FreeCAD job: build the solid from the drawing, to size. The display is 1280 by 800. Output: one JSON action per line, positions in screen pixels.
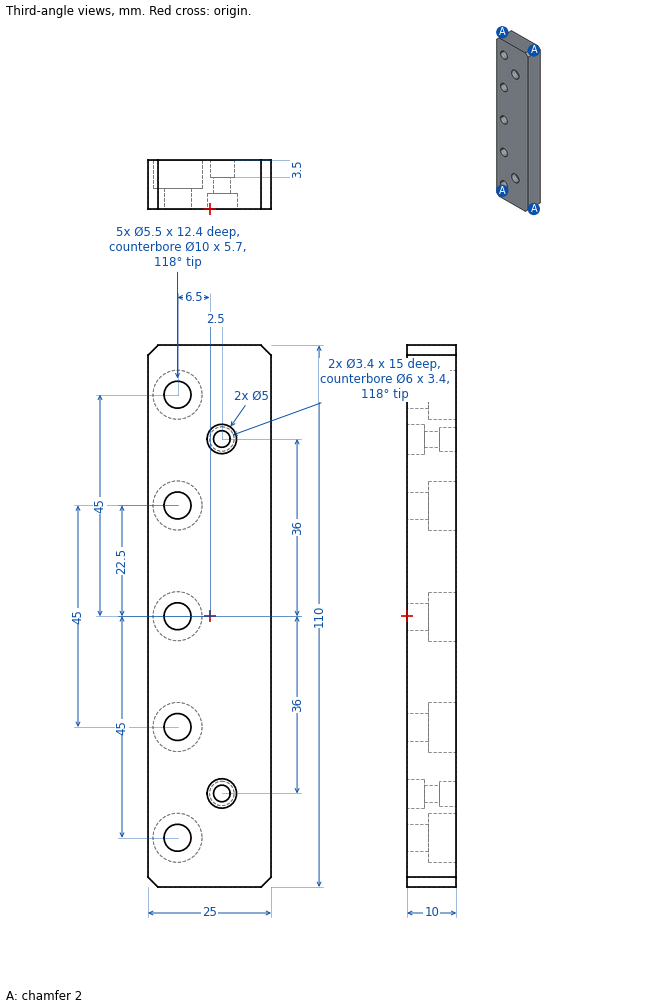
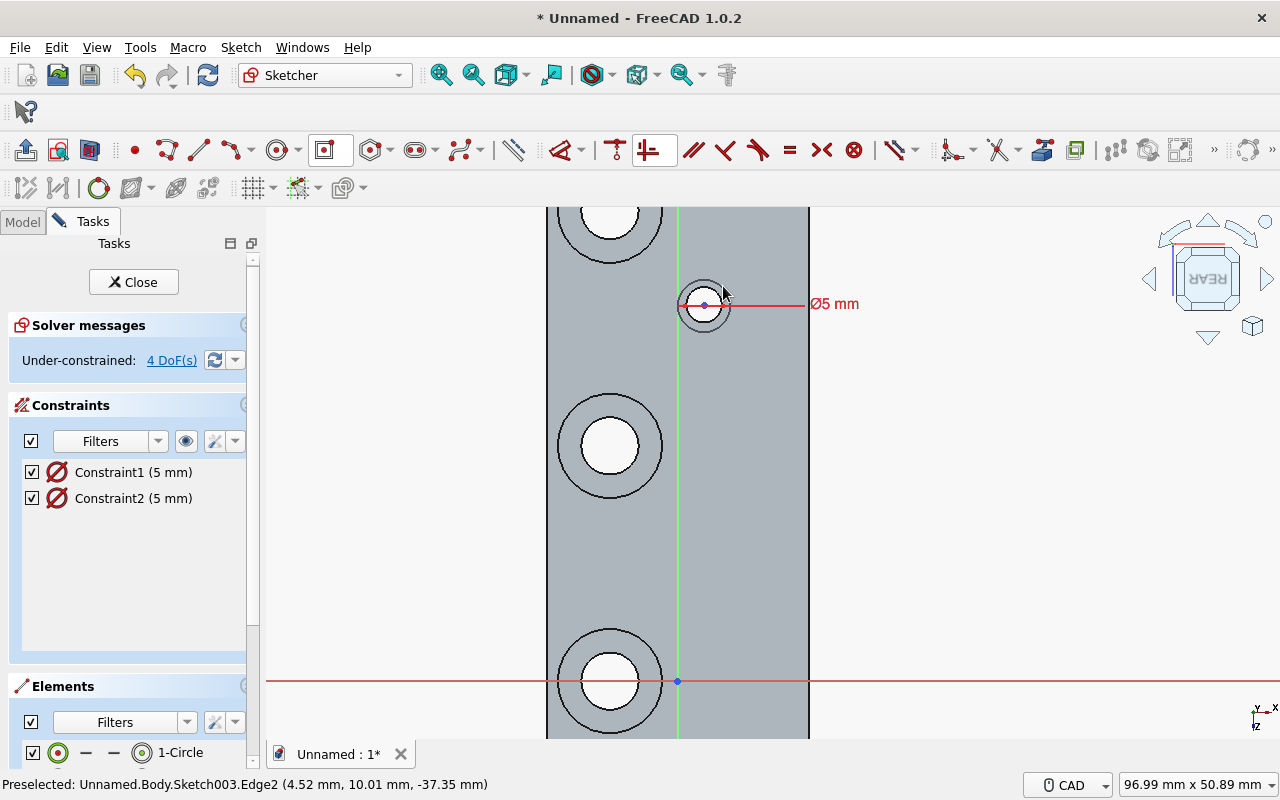
{"action": "scroll", "coordinate": [705, 303], "scroll_direction": "down", "scroll_amount": 4}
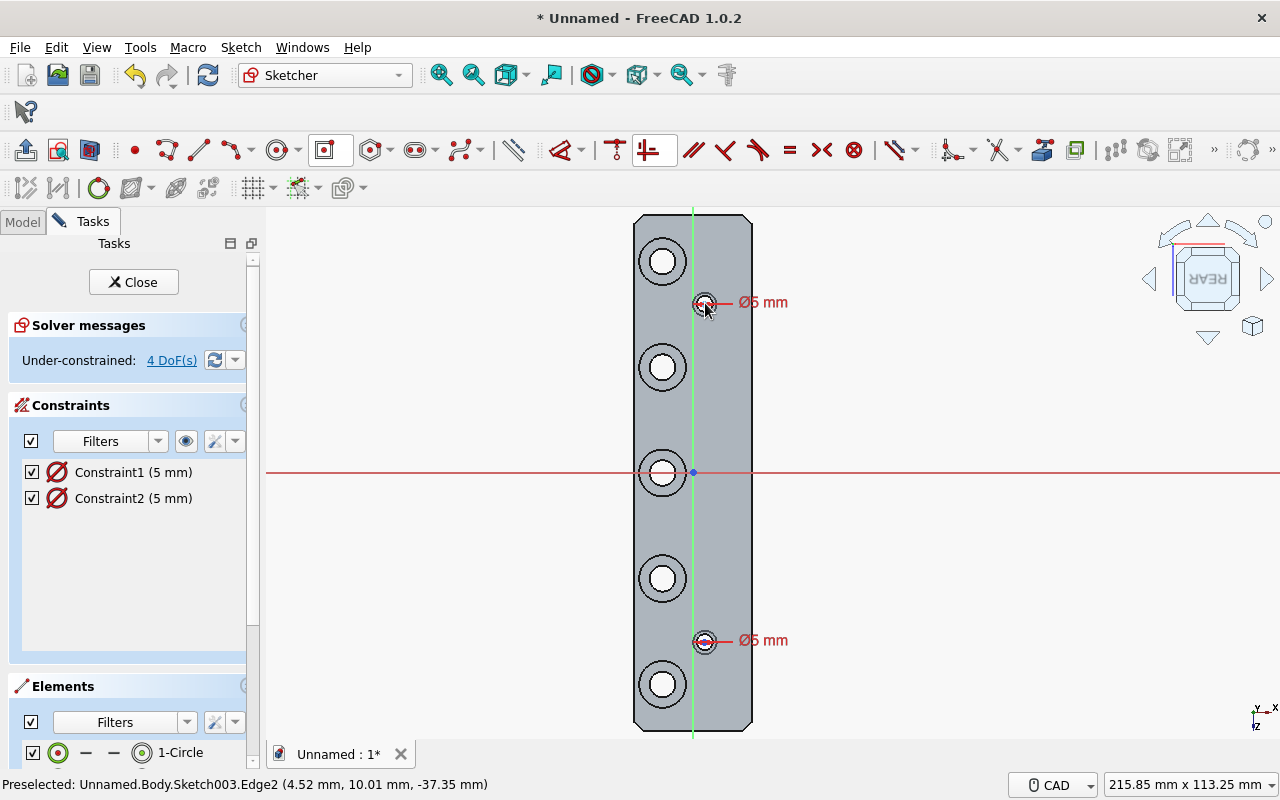
{"action": "left_click", "coordinate": [705, 642]}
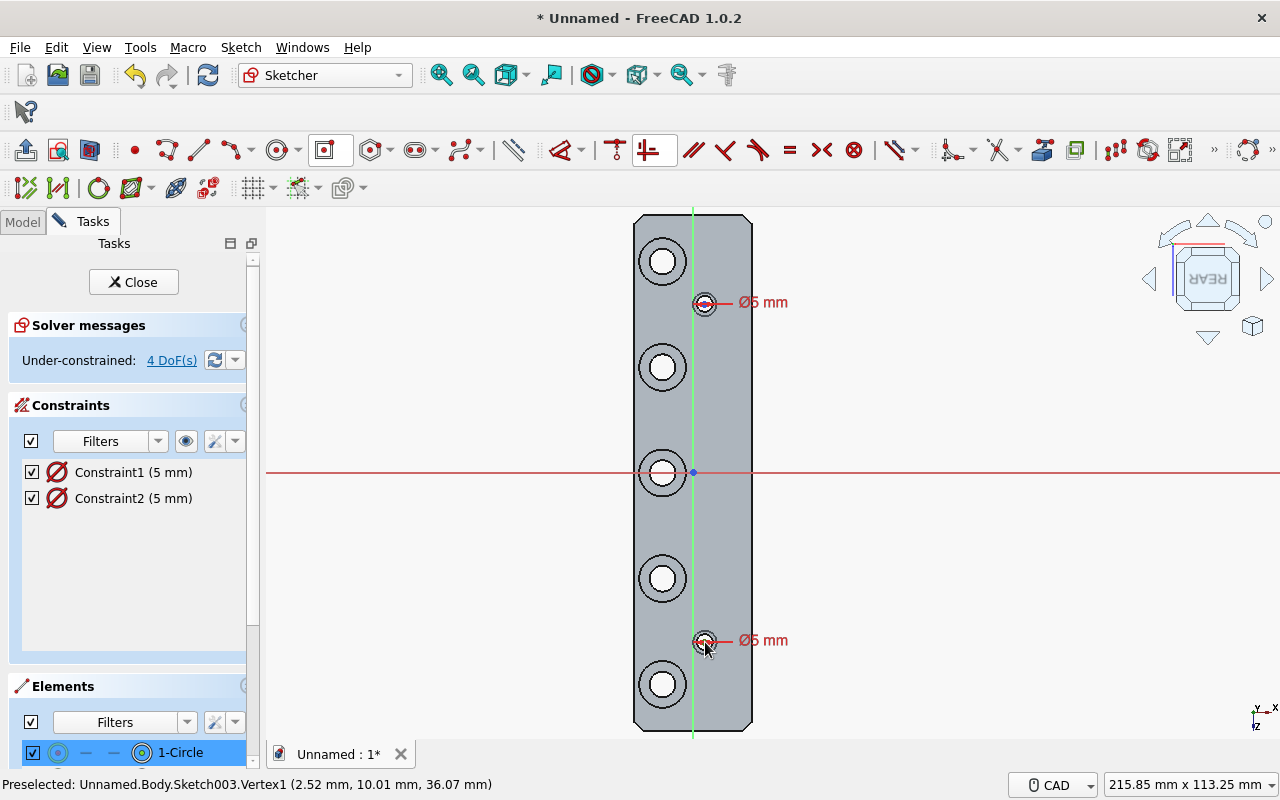
{"action": "left_click", "coordinate": [705, 304]}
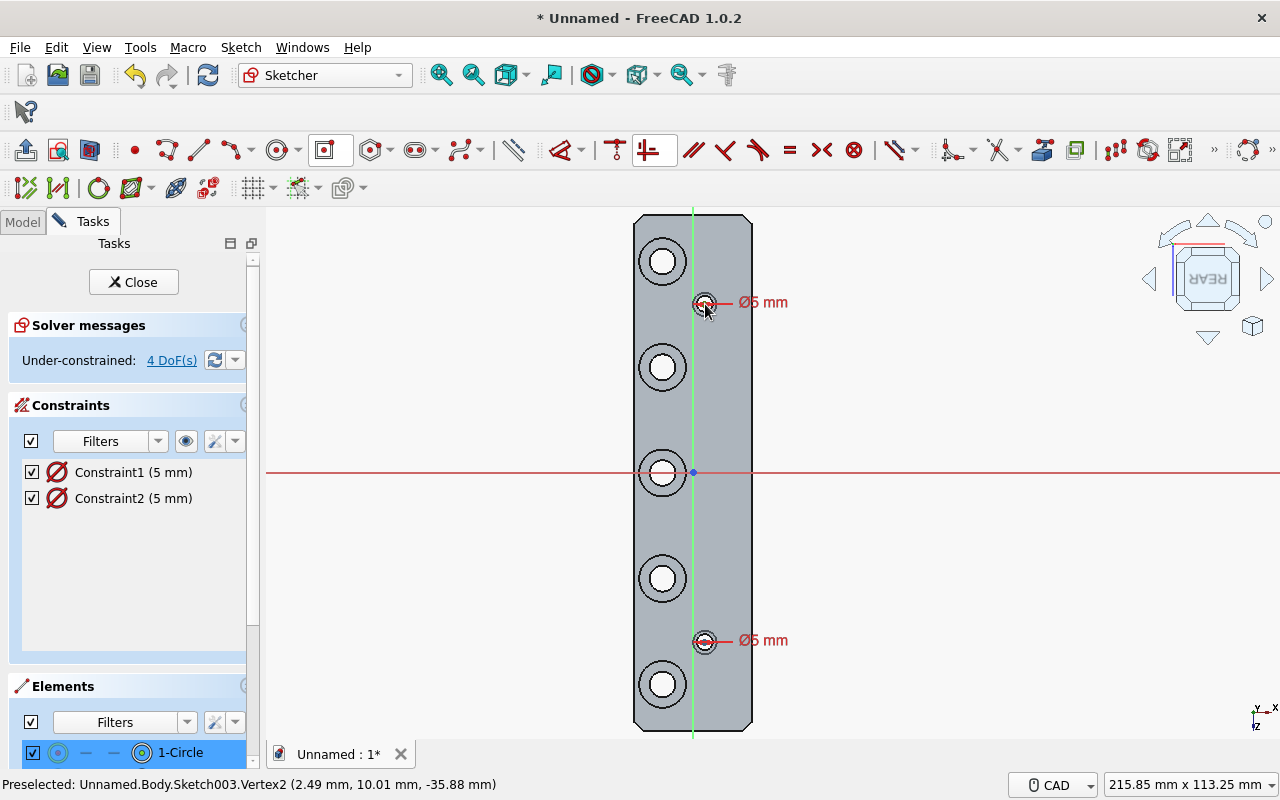
{"action": "key", "text": "v"}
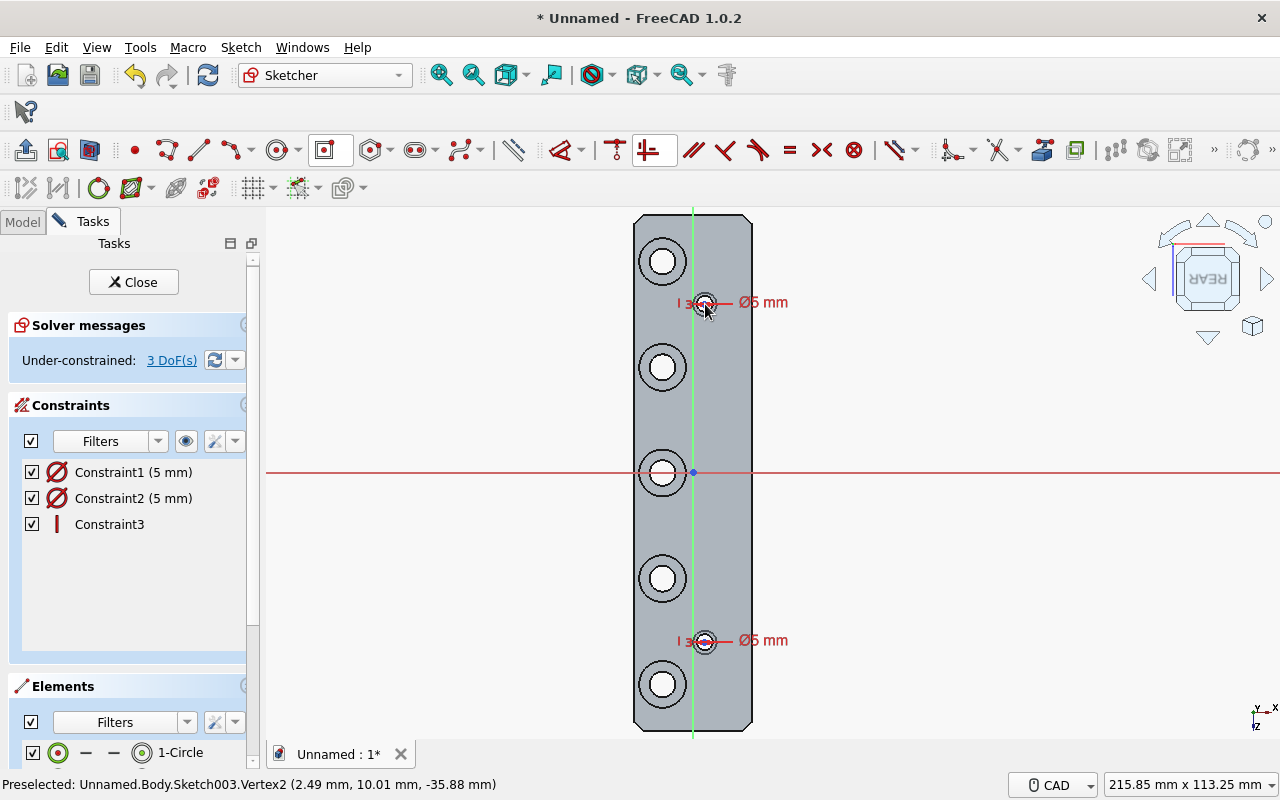
{"action": "left_click", "coordinate": [560, 150]}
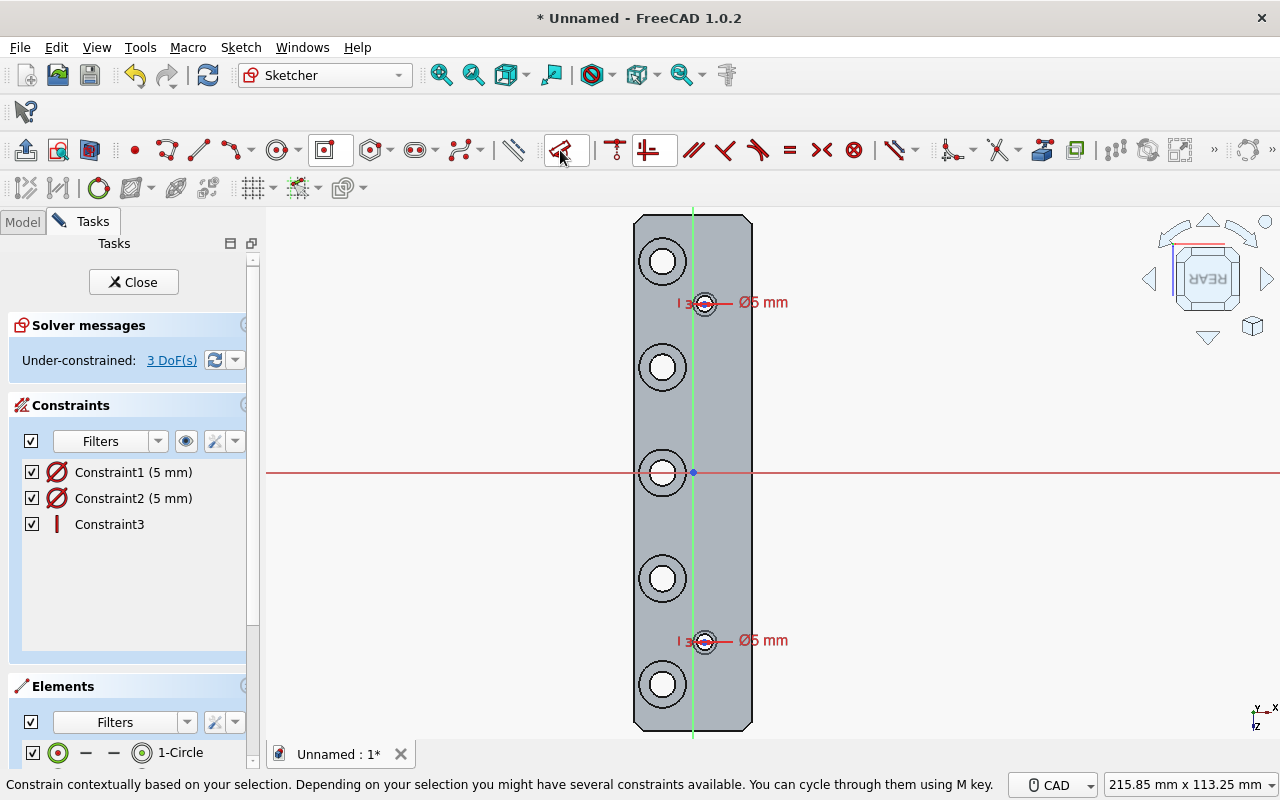
{"action": "left_click", "coordinate": [705, 642]}
{"action": "left_click", "coordinate": [659, 558]}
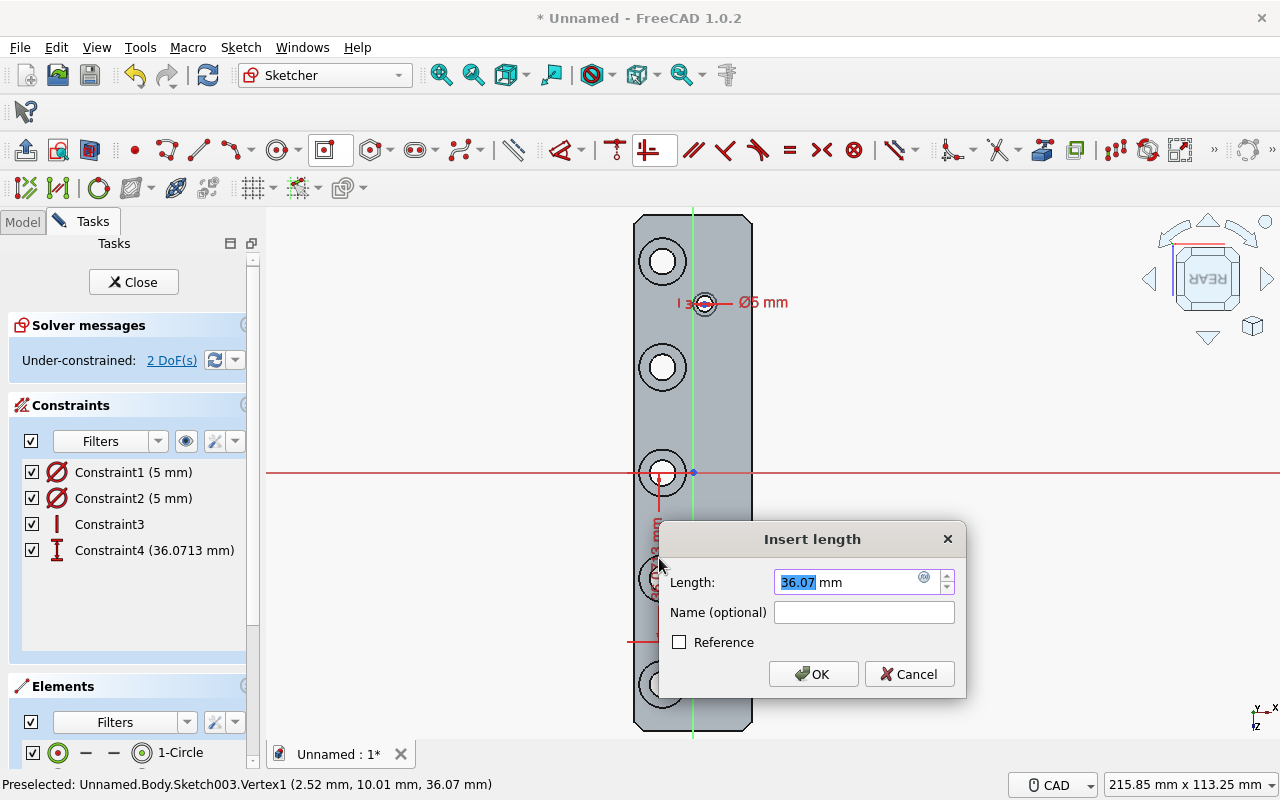
{"action": "type", "text": "36"}
{"action": "key", "text": "Return"}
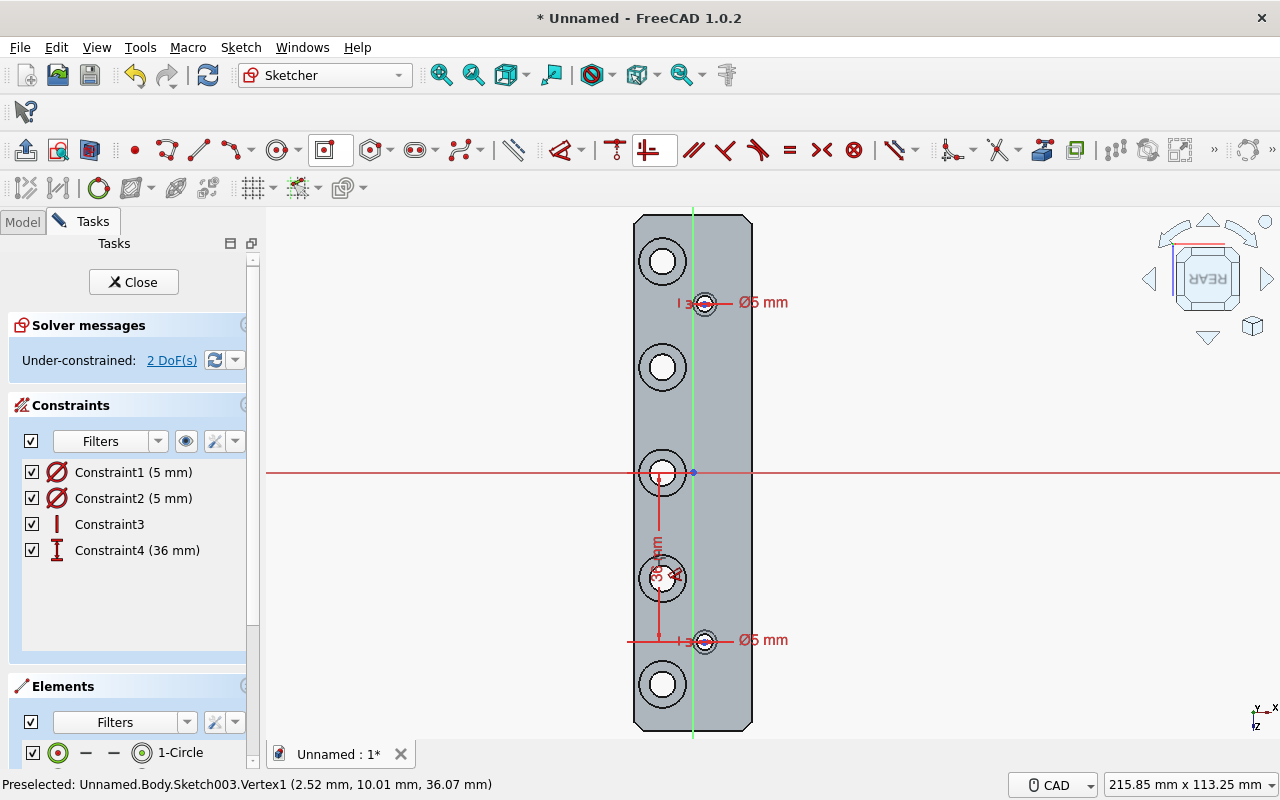
{"action": "left_click", "coordinate": [705, 304]}
{"action": "left_click", "coordinate": [659, 389]}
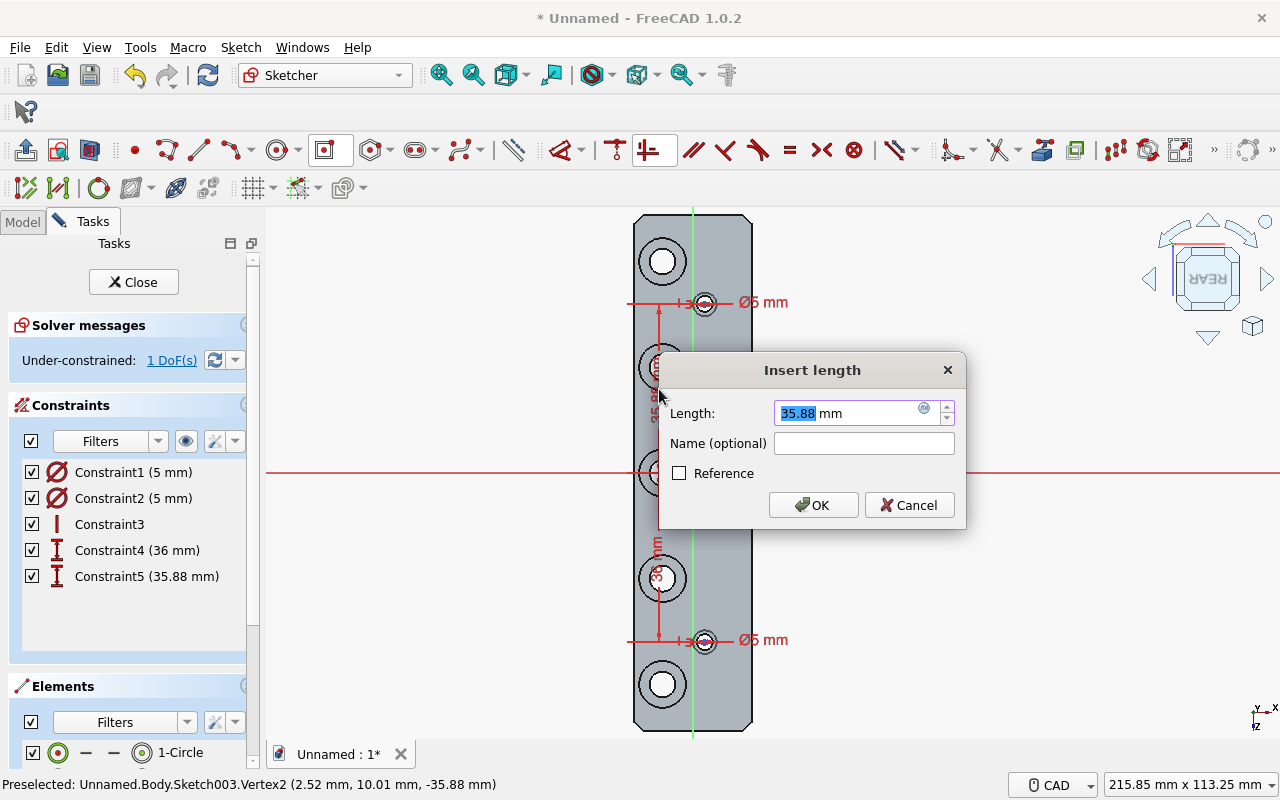
{"action": "type", "text": "36"}
{"action": "key", "text": "Return"}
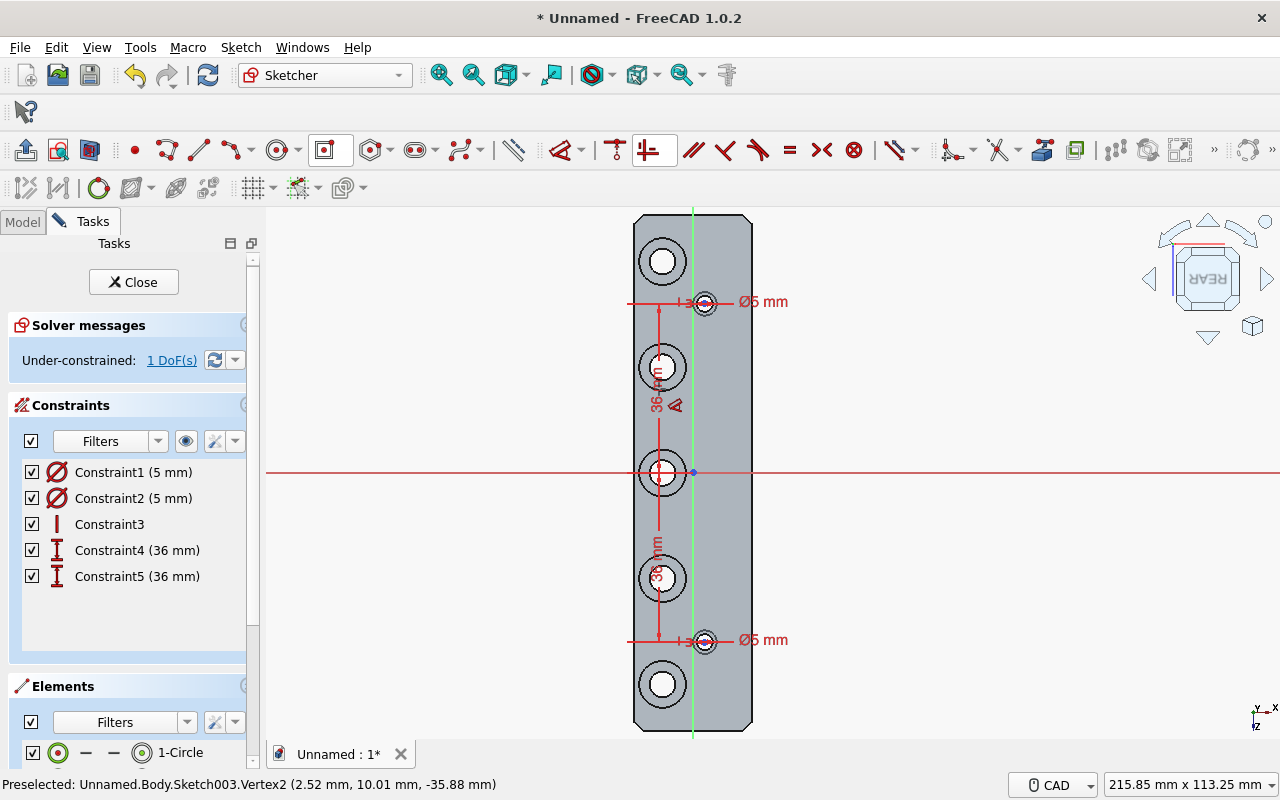
{"action": "scroll", "coordinate": [705, 642], "scroll_direction": "up", "scroll_amount": 7}